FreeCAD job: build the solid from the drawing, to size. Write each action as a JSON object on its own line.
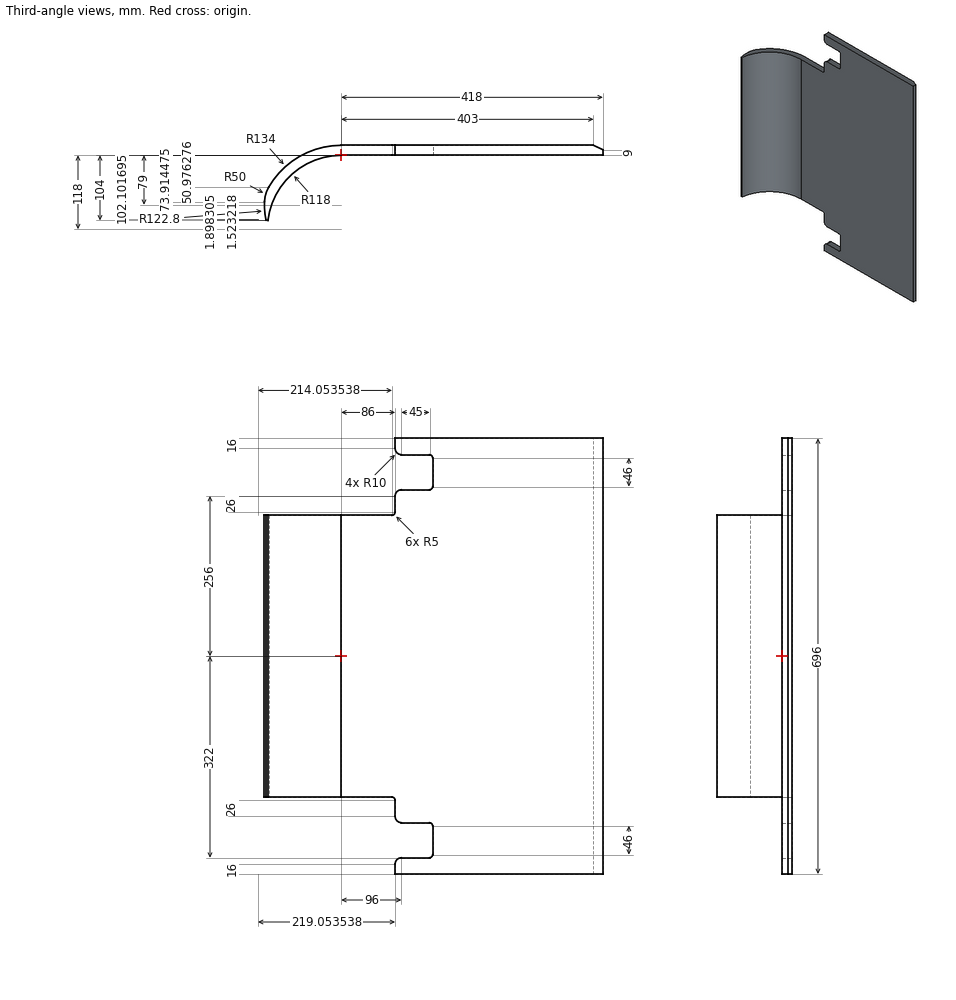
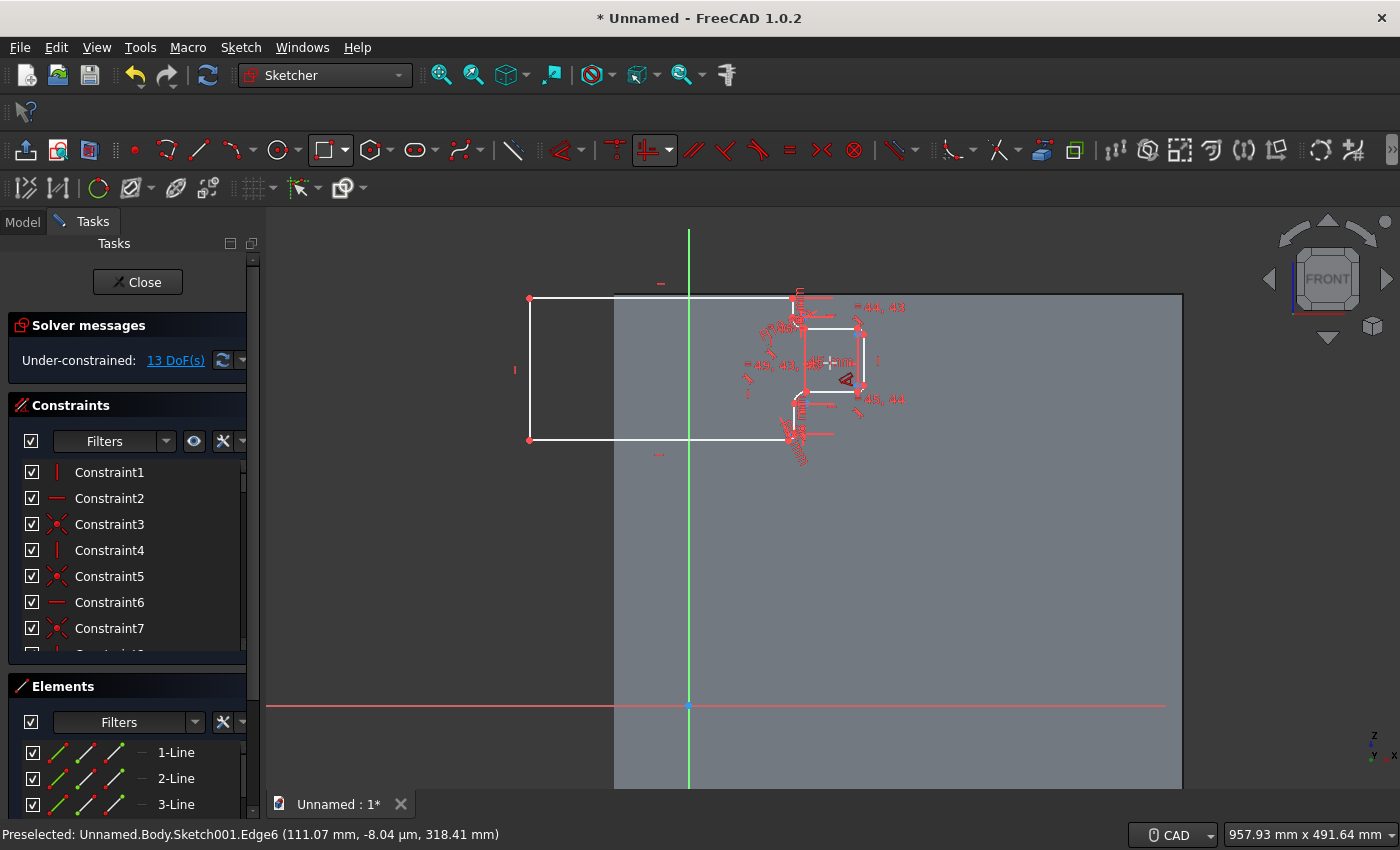
{"action": "left_click", "coordinate": [864, 350]}
{"action": "left_click", "coordinate": [898, 342]}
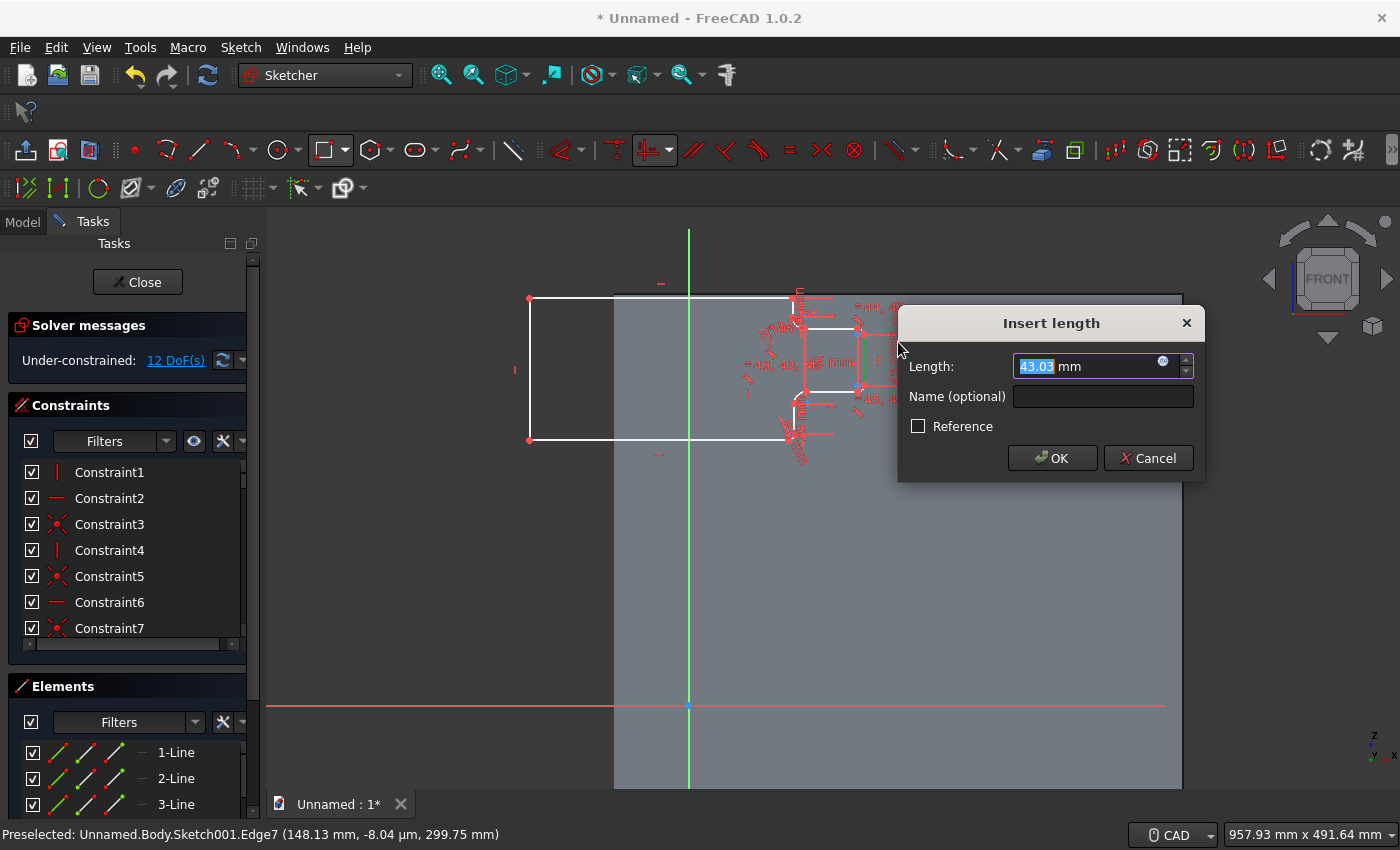
{"action": "type", "text": "46"}
{"action": "key", "text": "Return"}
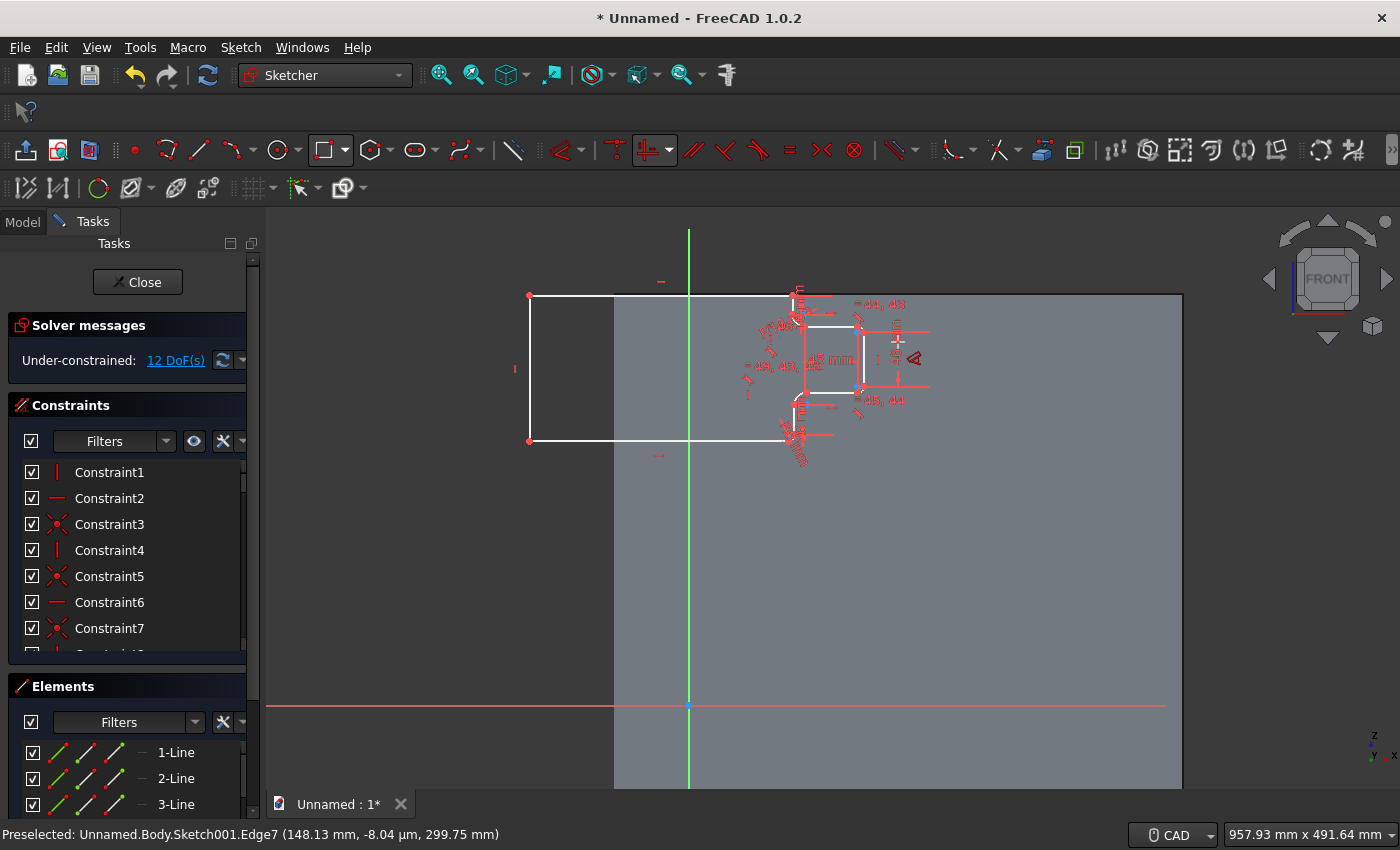
{"action": "left_click", "coordinate": [842, 393]}
{"action": "left_click", "coordinate": [832, 475]}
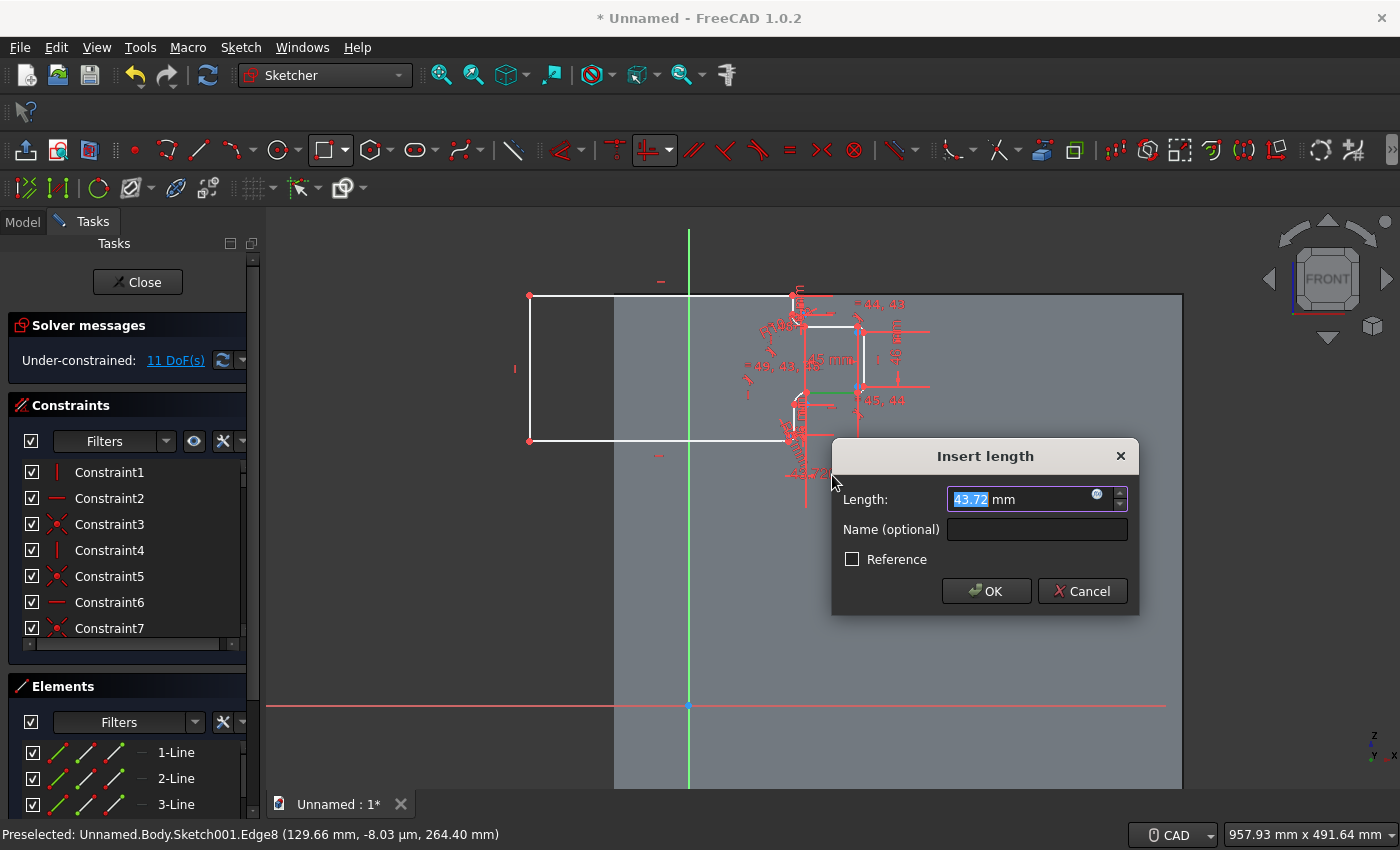
{"action": "type", "text": "45"}
{"action": "key", "text": "Return"}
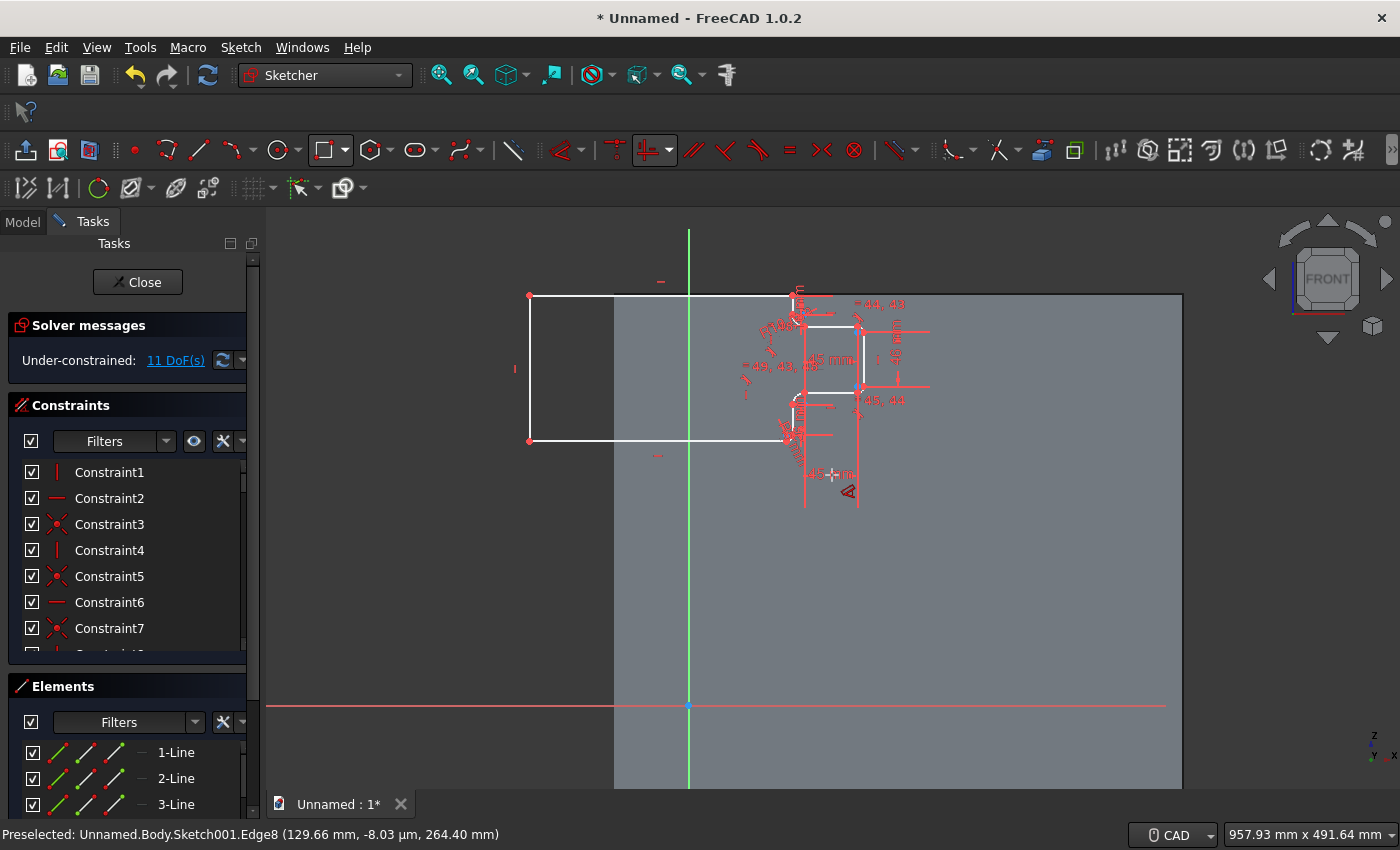
{"action": "scroll", "coordinate": [820, 328], "scroll_direction": "down", "scroll_amount": 4}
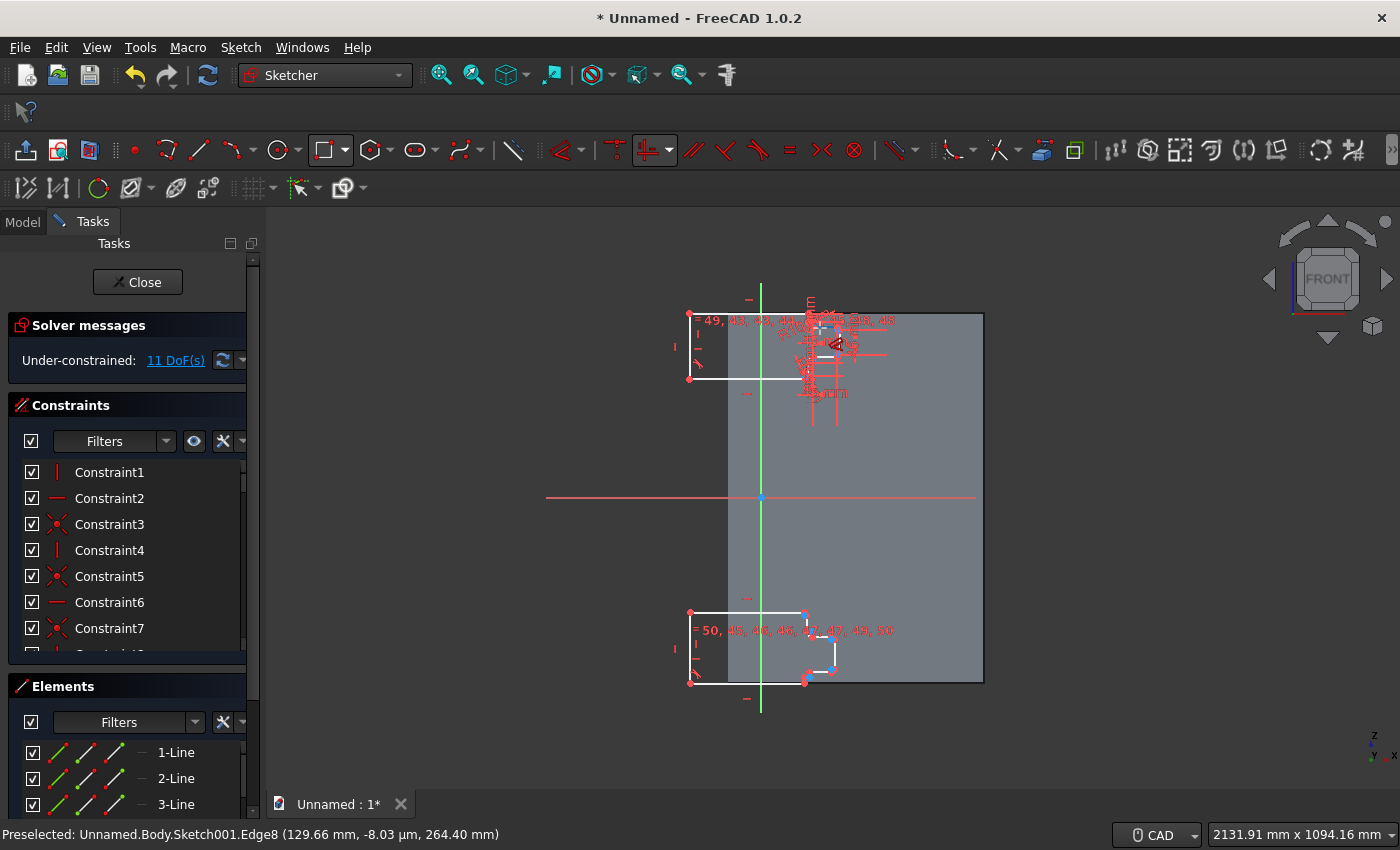
{"action": "scroll", "coordinate": [825, 672], "scroll_direction": "up", "scroll_amount": 4}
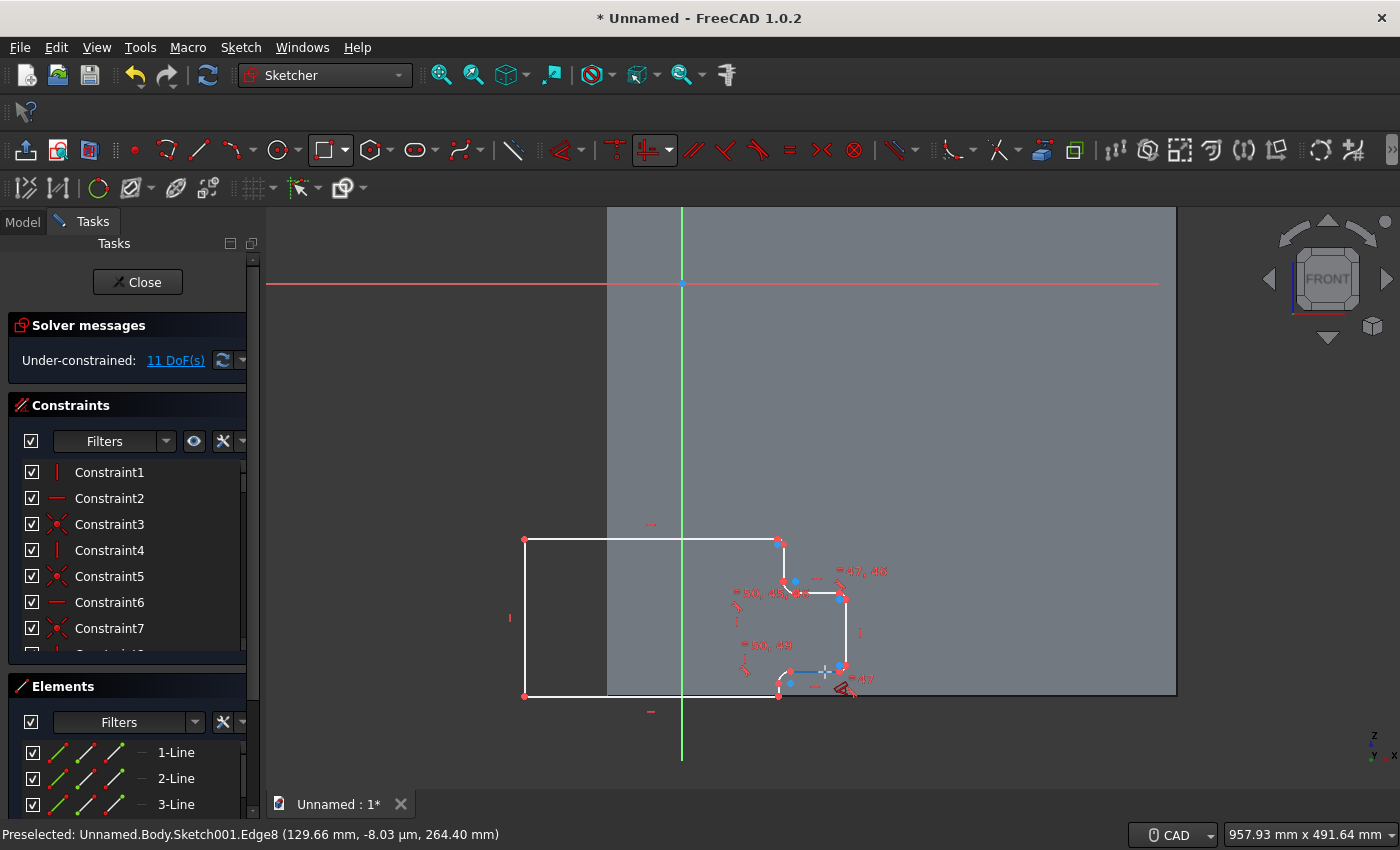
{"action": "left_click", "coordinate": [825, 672]}
{"action": "left_click", "coordinate": [815, 706]}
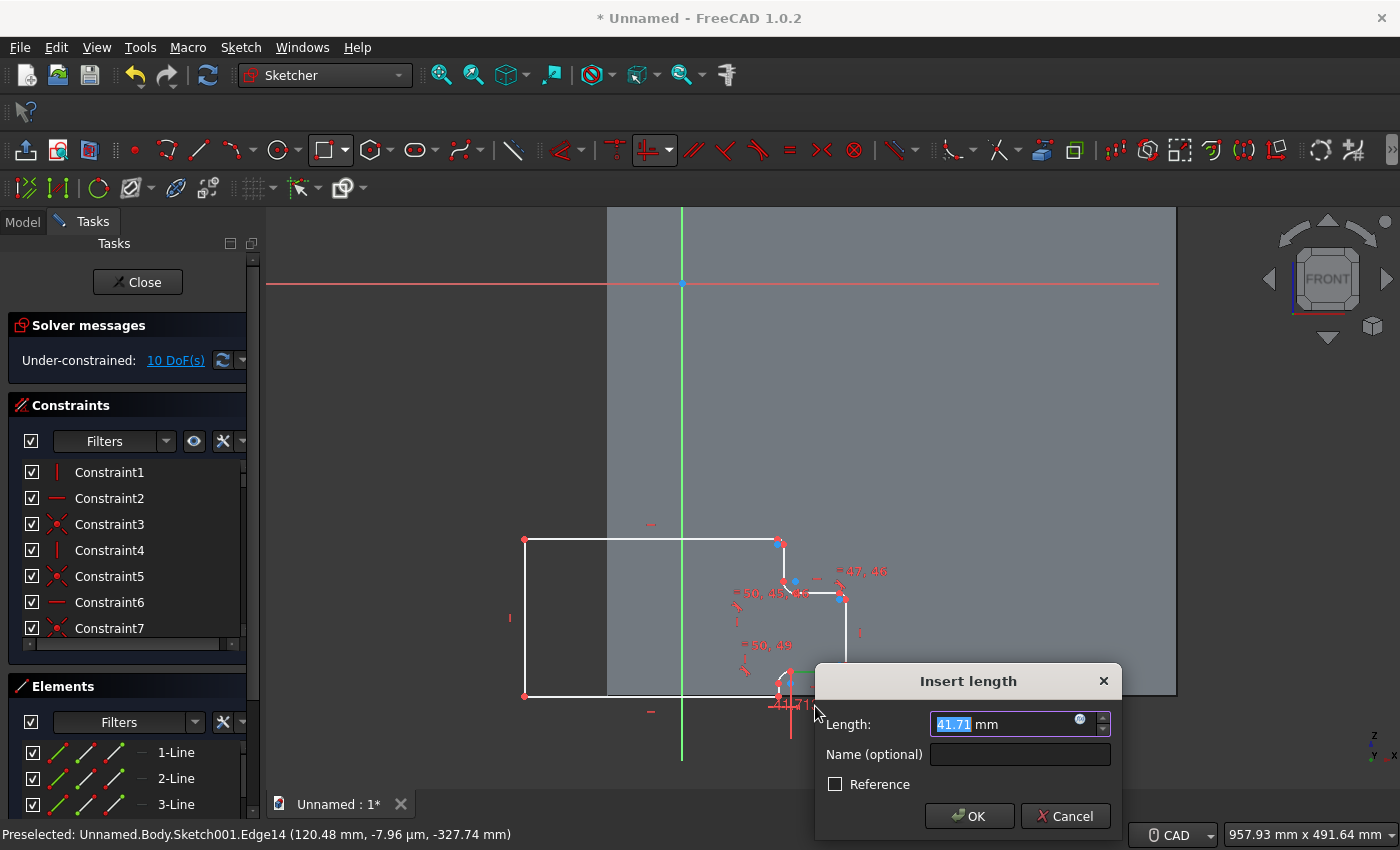
{"action": "type", "text": "45"}
{"action": "key", "text": "Return"}